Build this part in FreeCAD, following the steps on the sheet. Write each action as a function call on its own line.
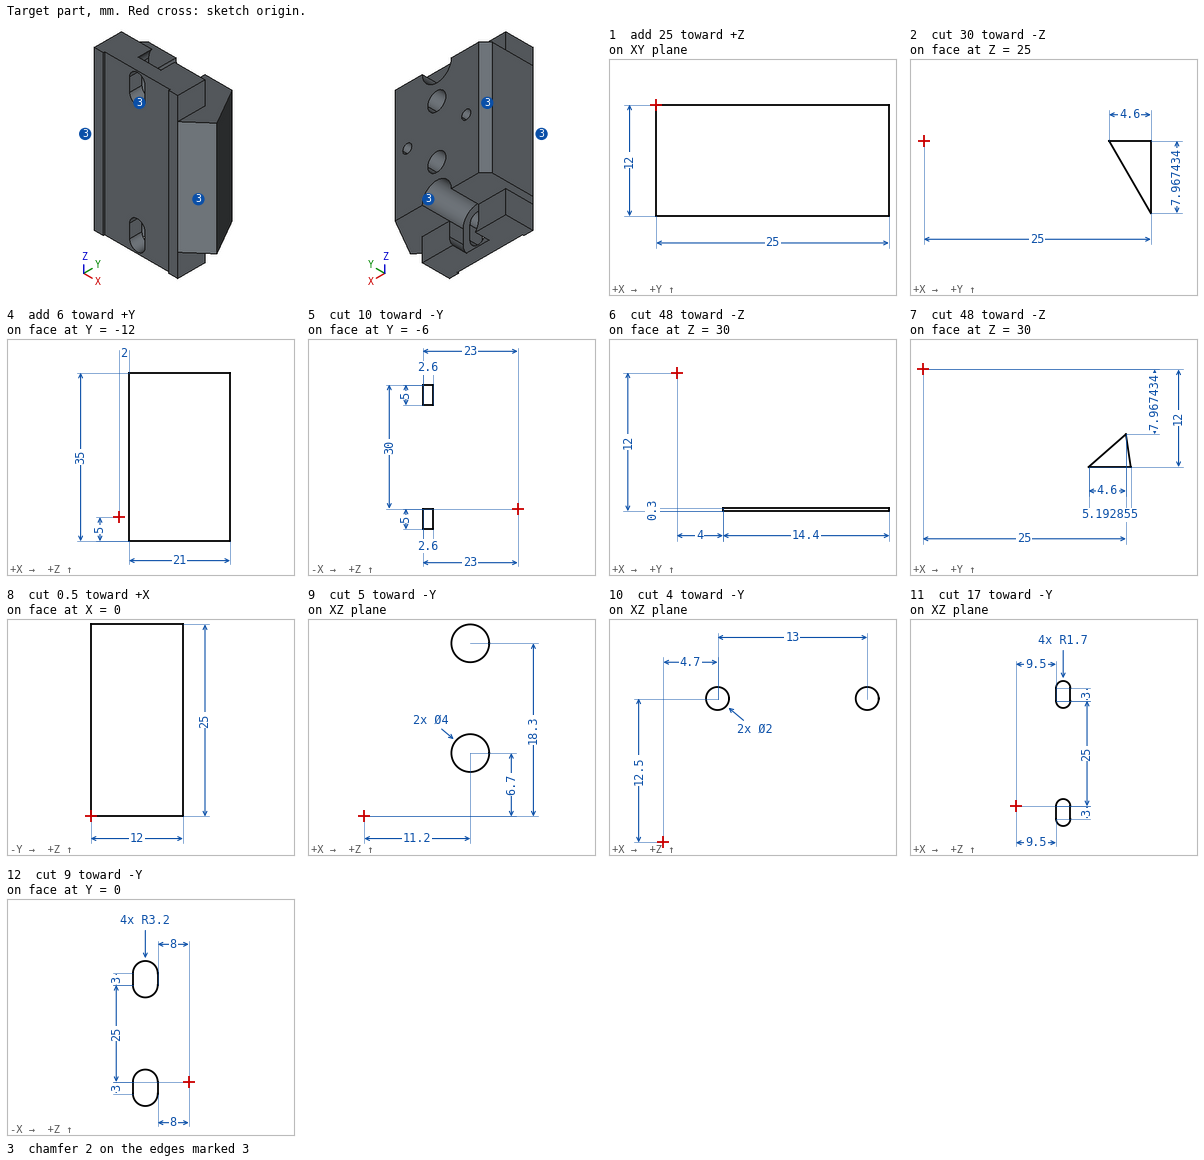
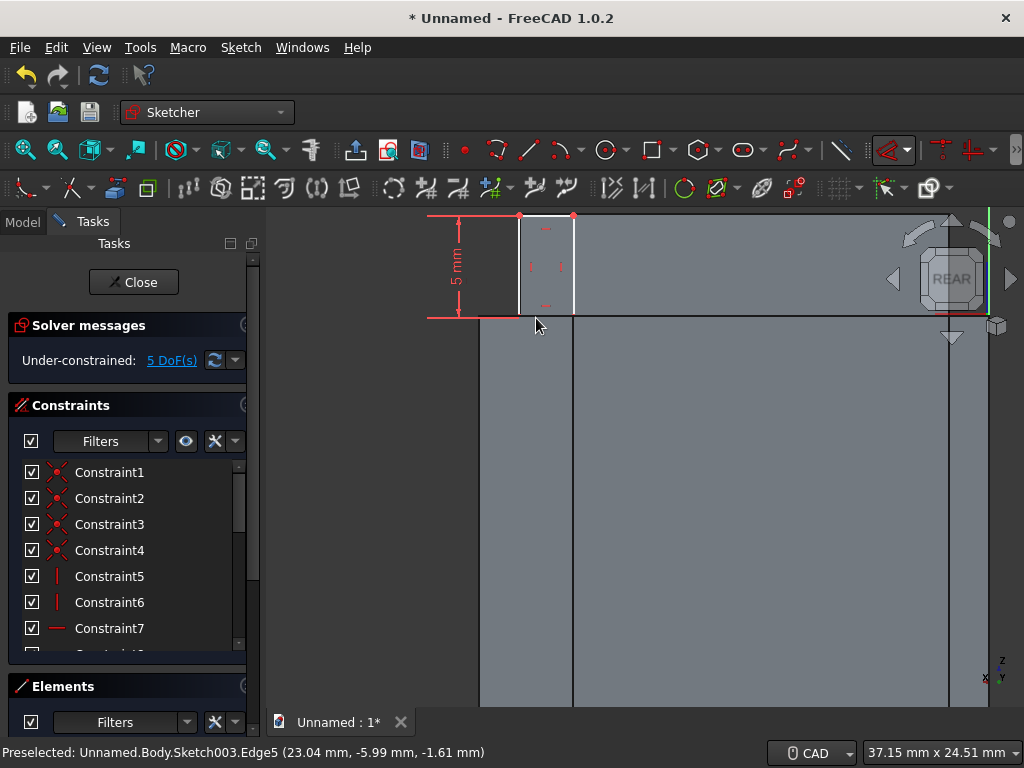
click(536, 318)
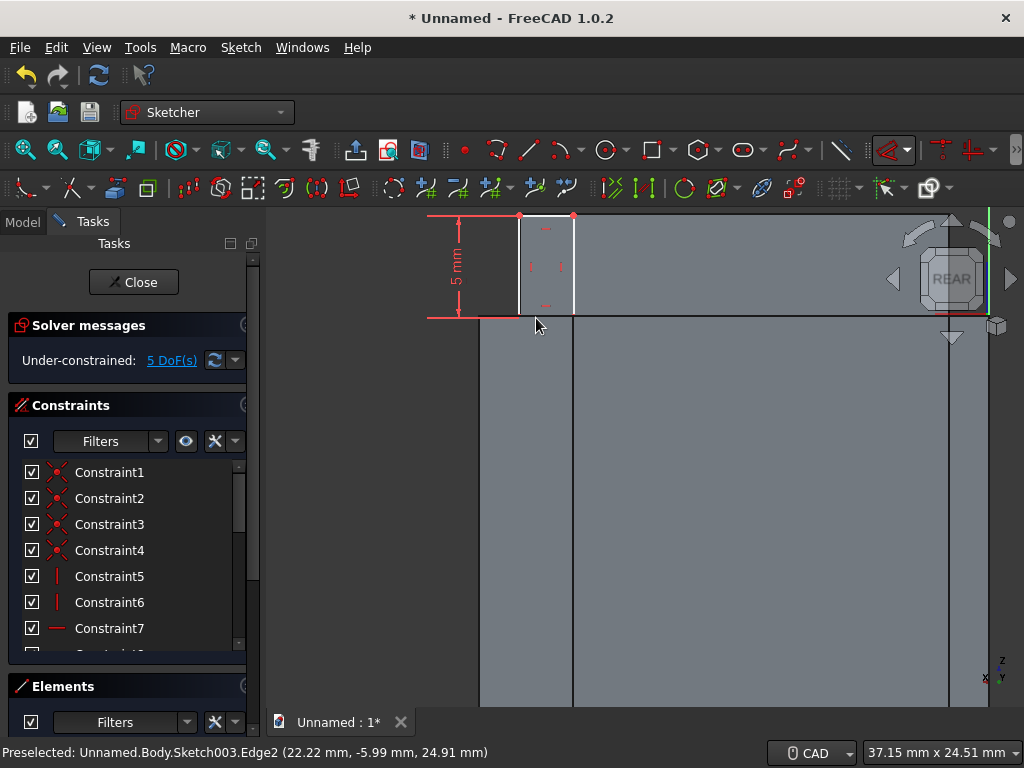
key(l)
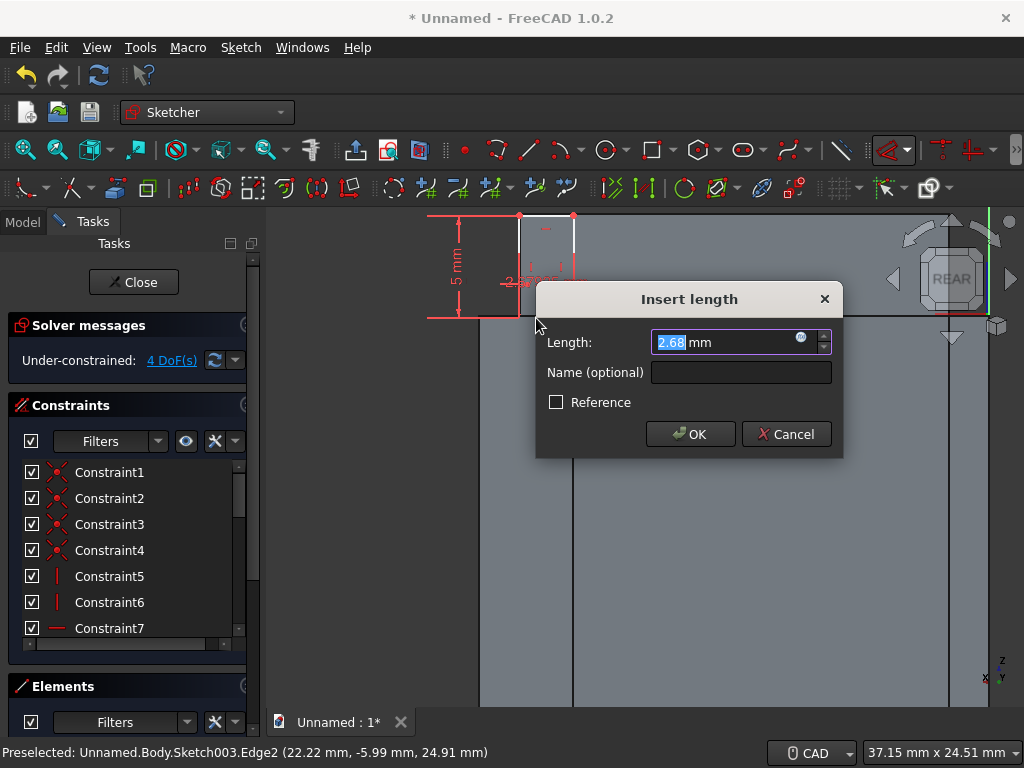
text(2.6)
key(Return)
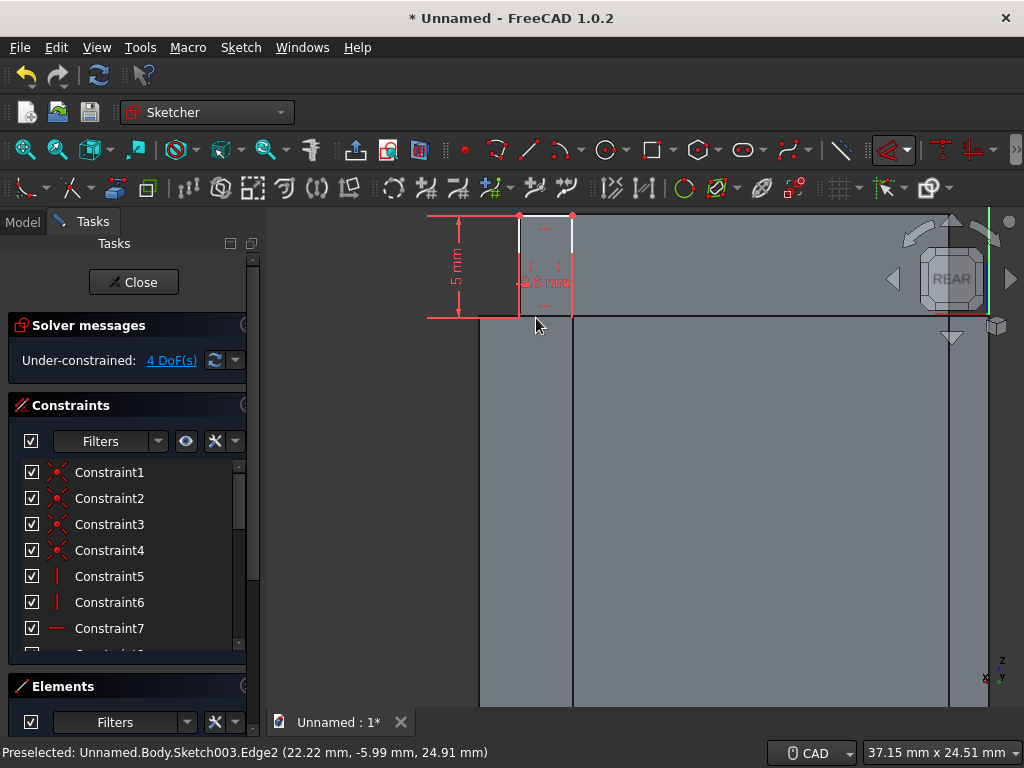
scroll(431, 364, down, 4)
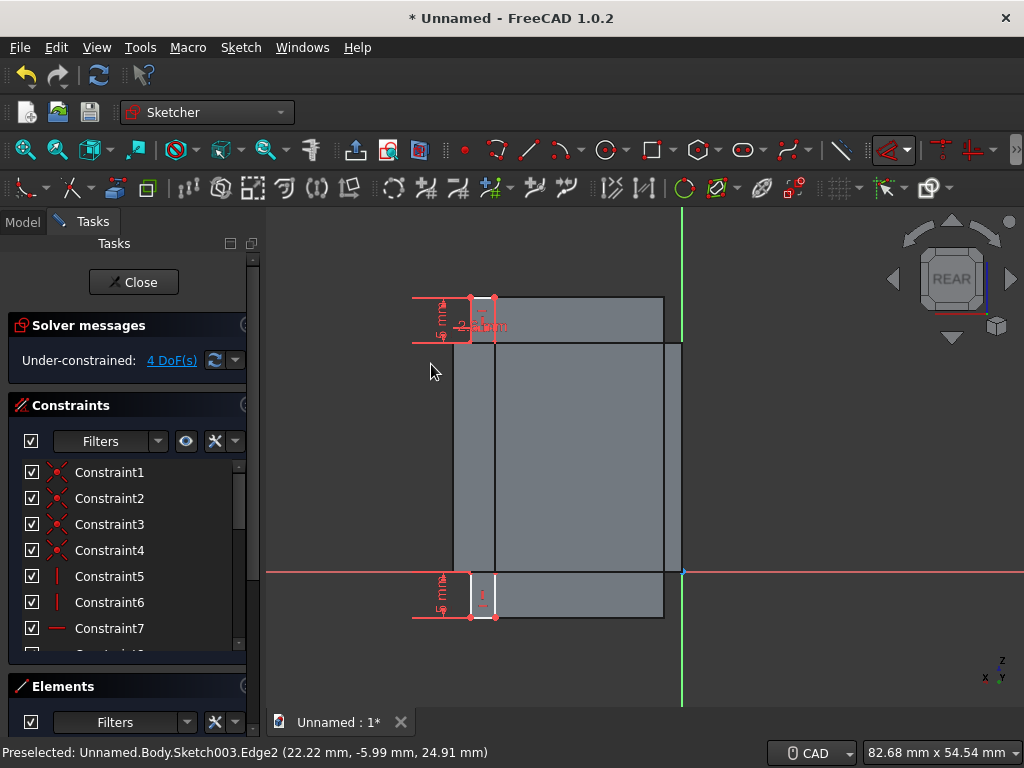
scroll(478, 618, up, 4)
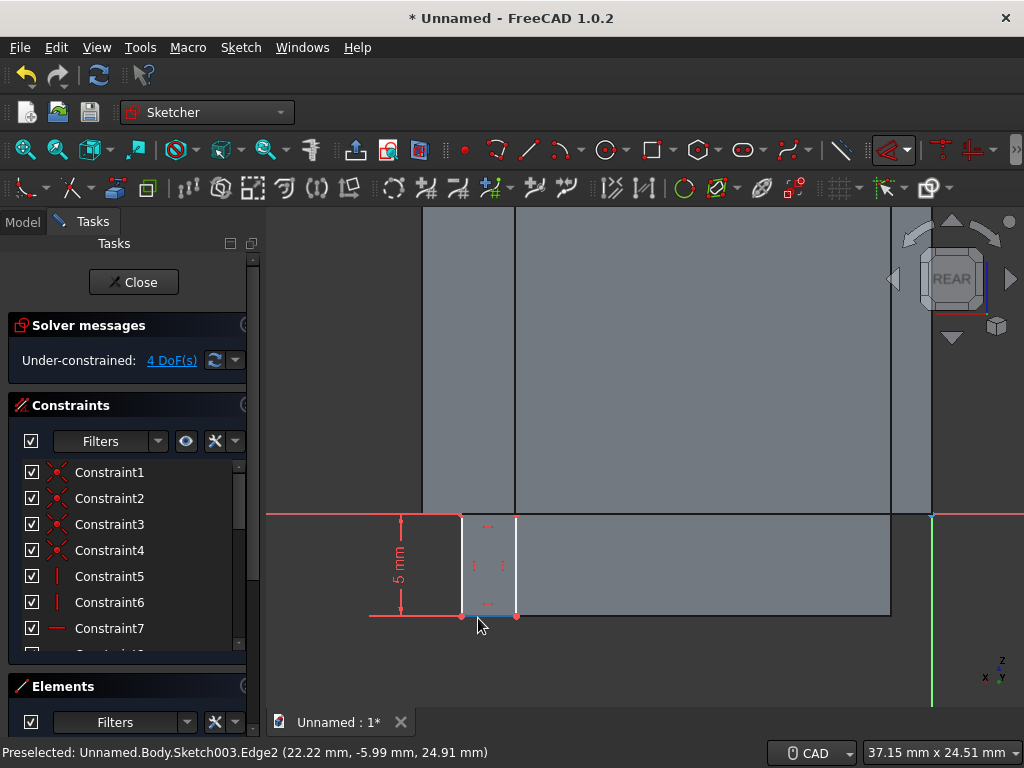
click(478, 616)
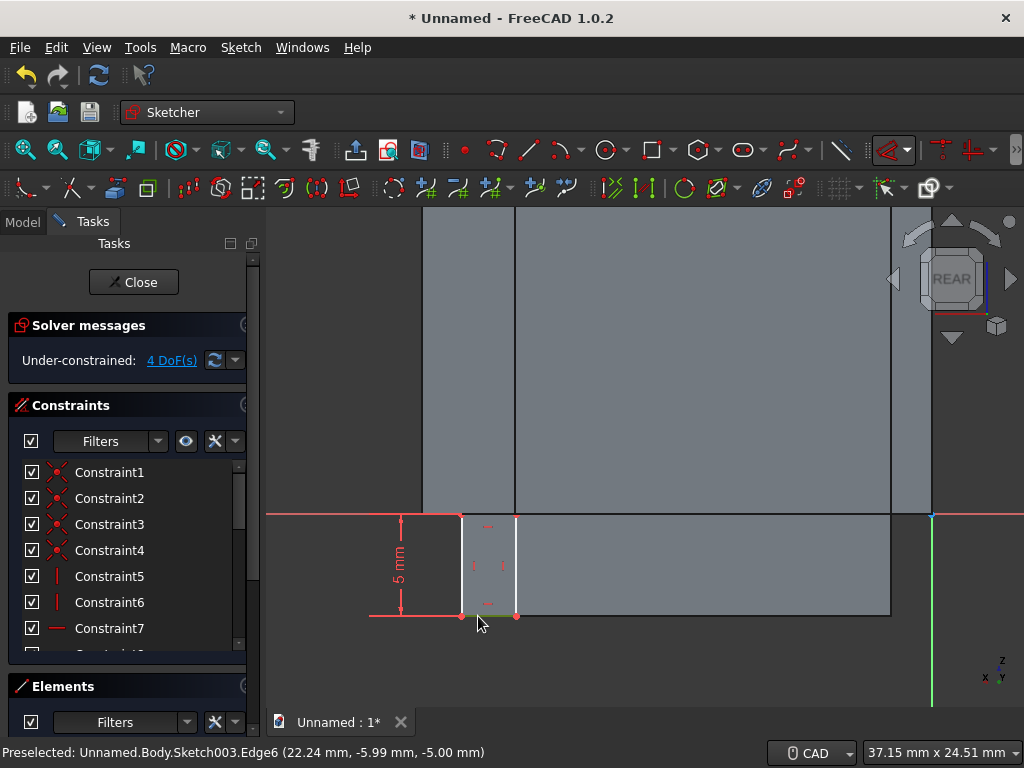
key(l)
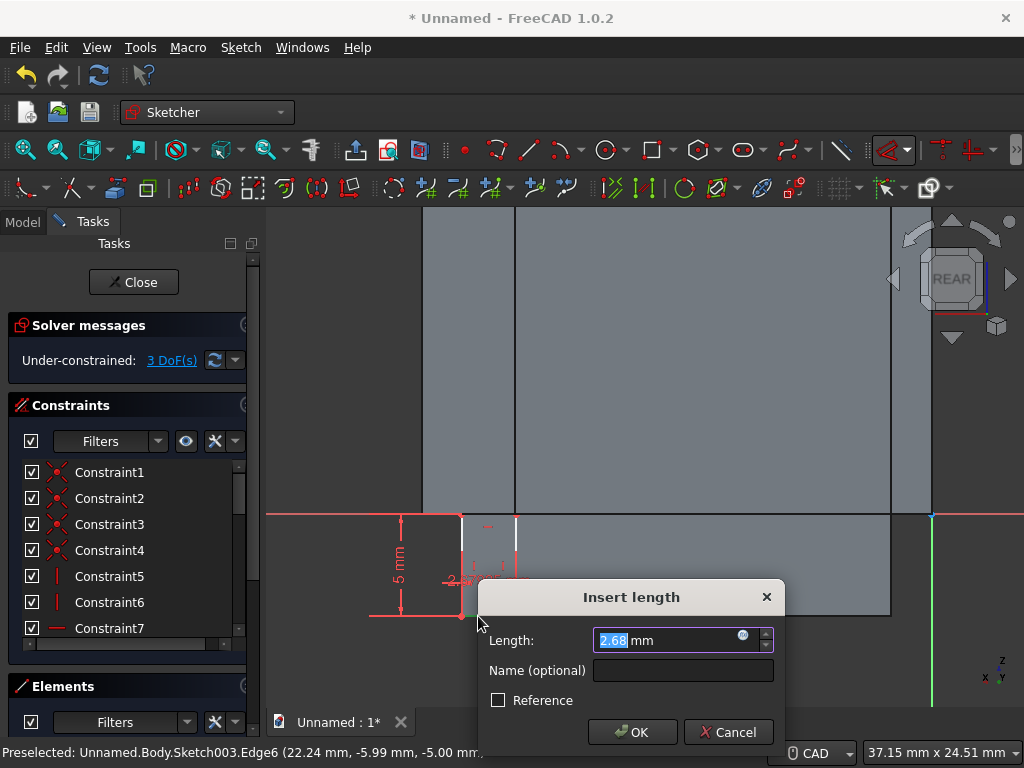
text(2.6)
key(Return)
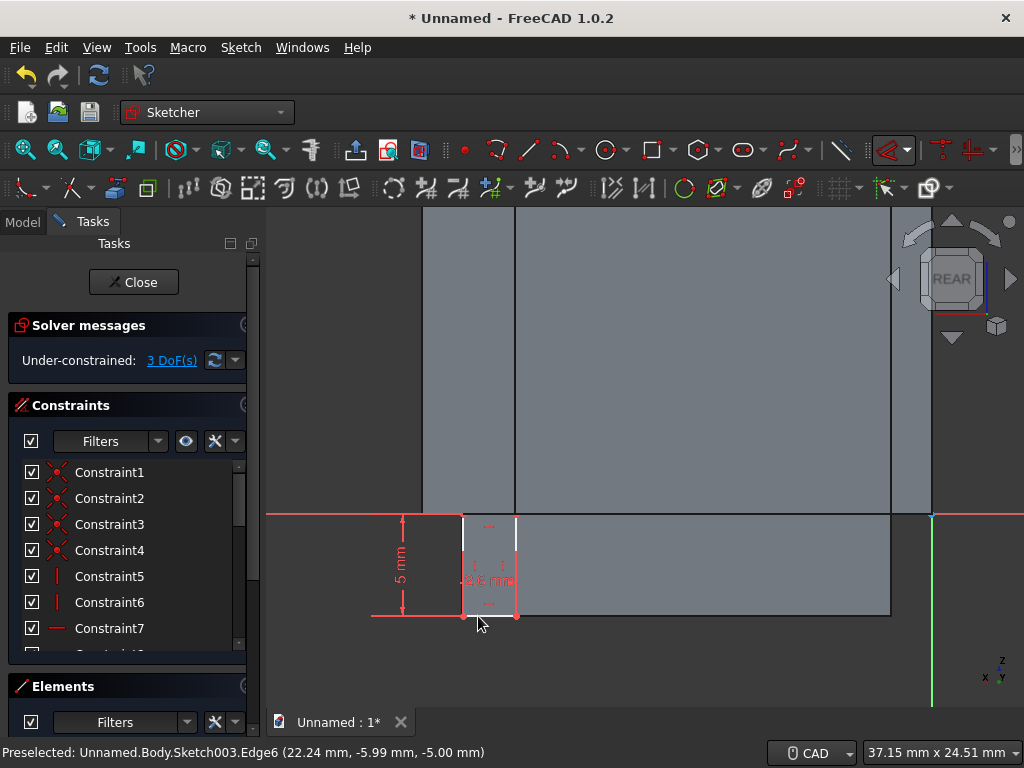
scroll(478, 618, down, 4)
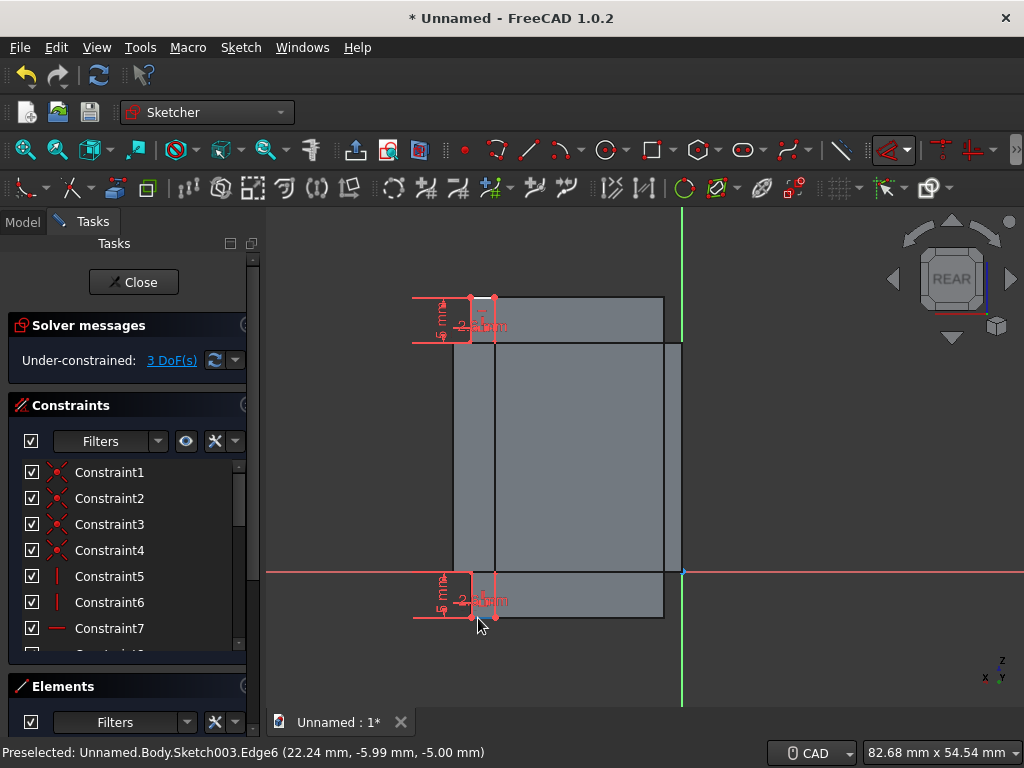
click(471, 298)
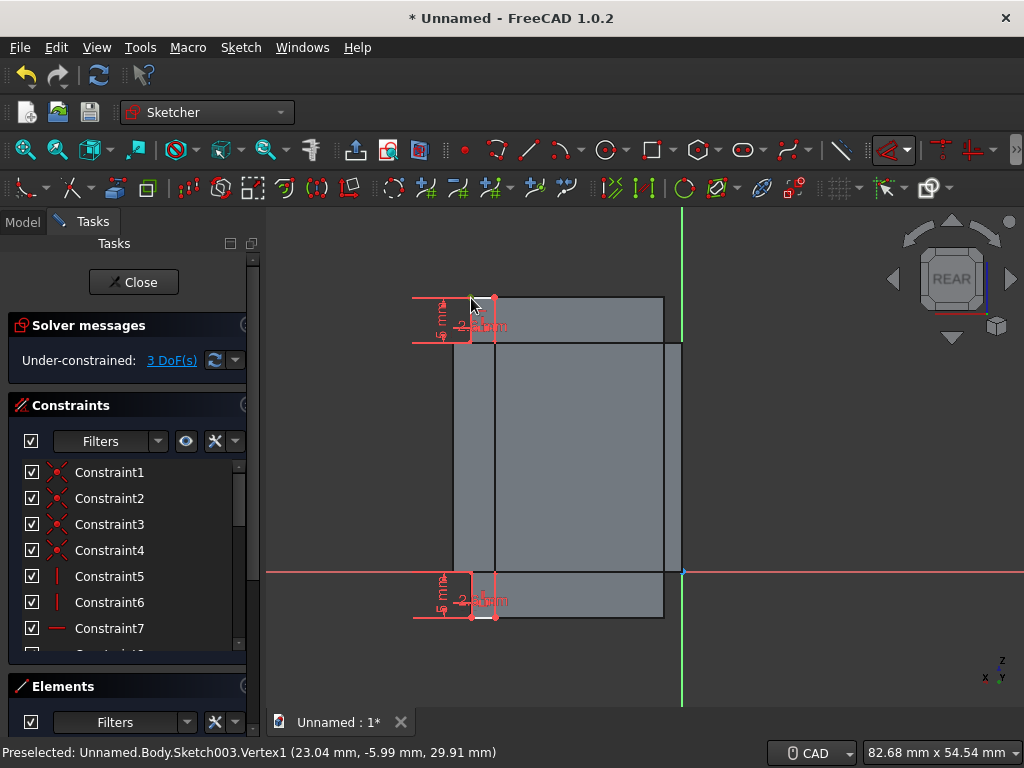
key(l)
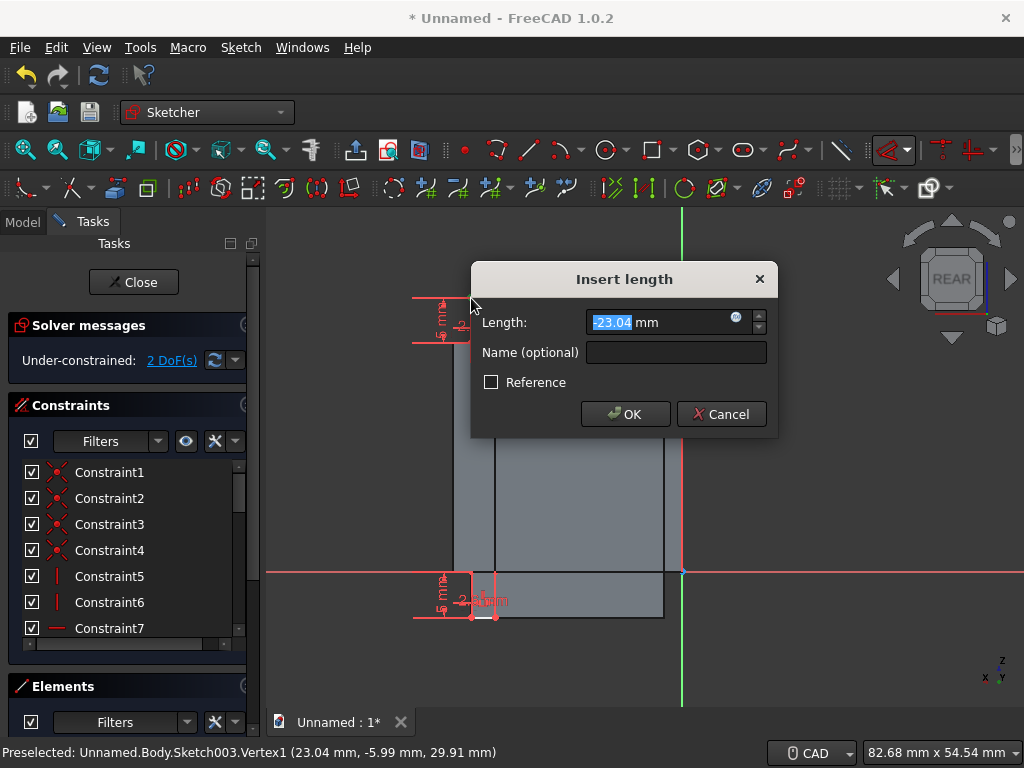
text(-23)
key(Return)